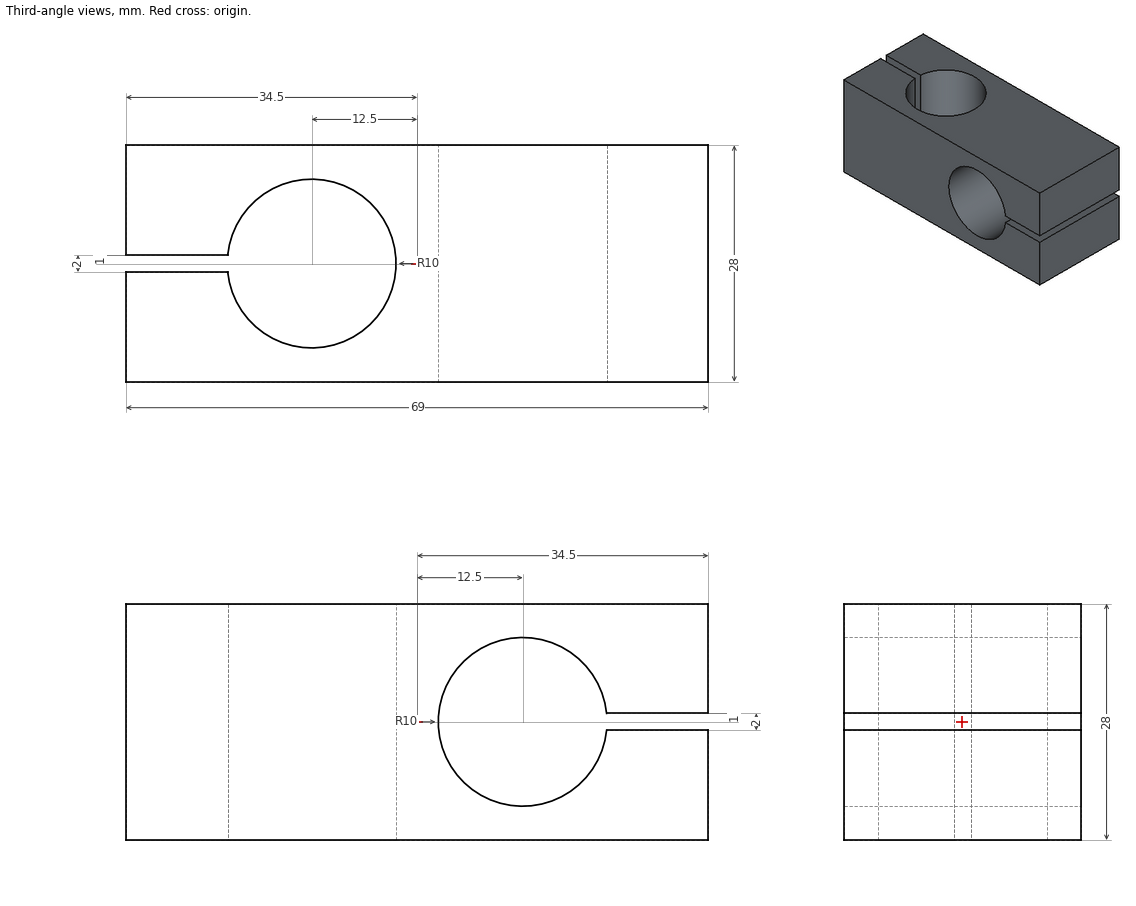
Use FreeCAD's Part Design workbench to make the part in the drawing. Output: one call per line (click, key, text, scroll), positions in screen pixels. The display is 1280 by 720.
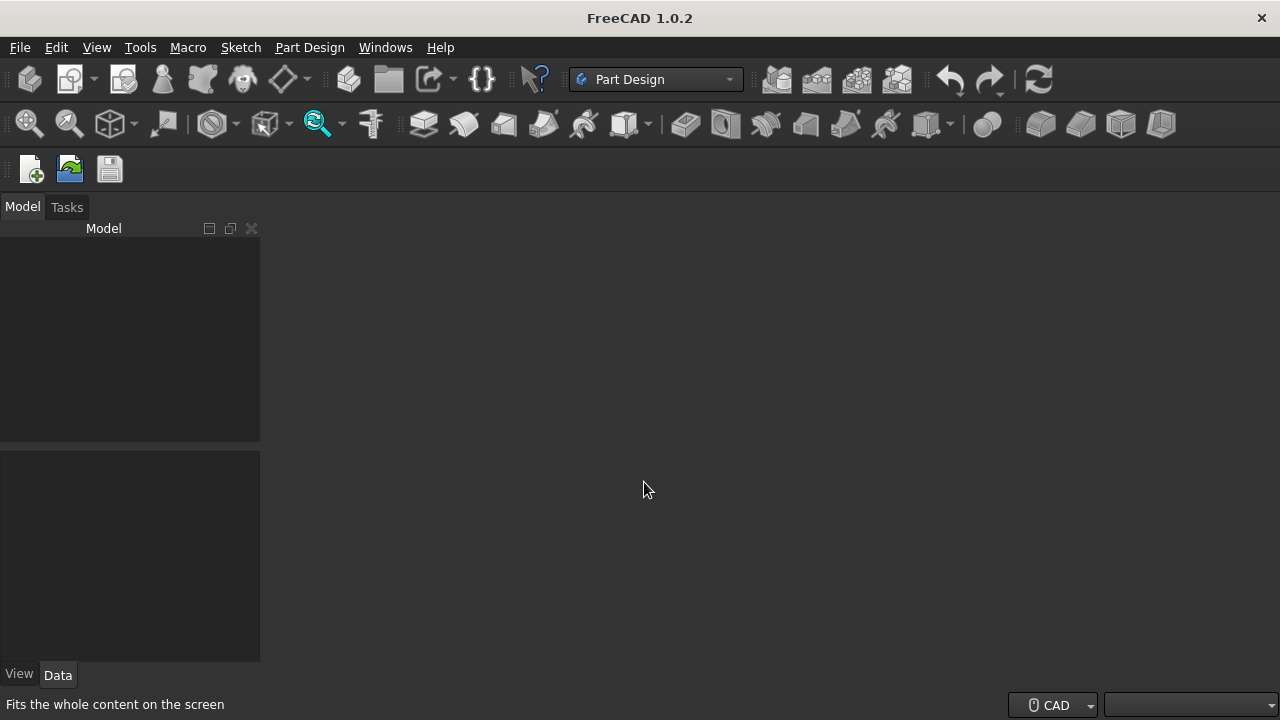
key(ctrl+n)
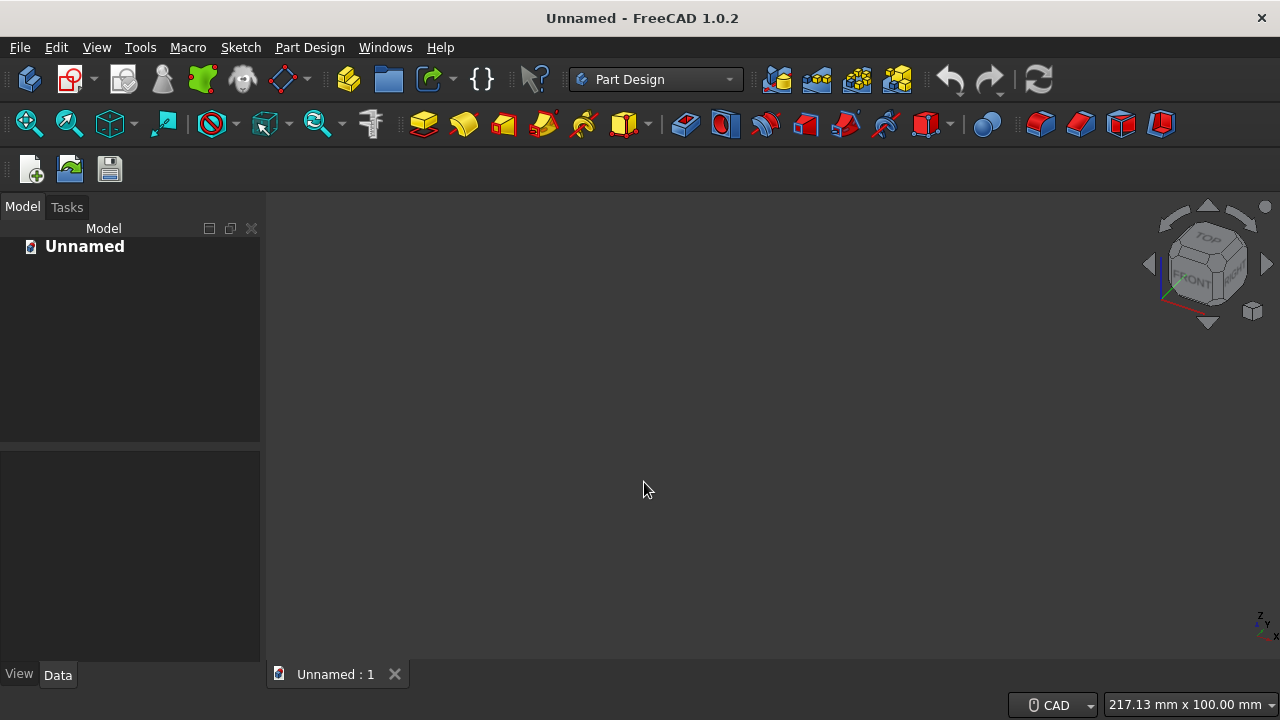
click(70, 80)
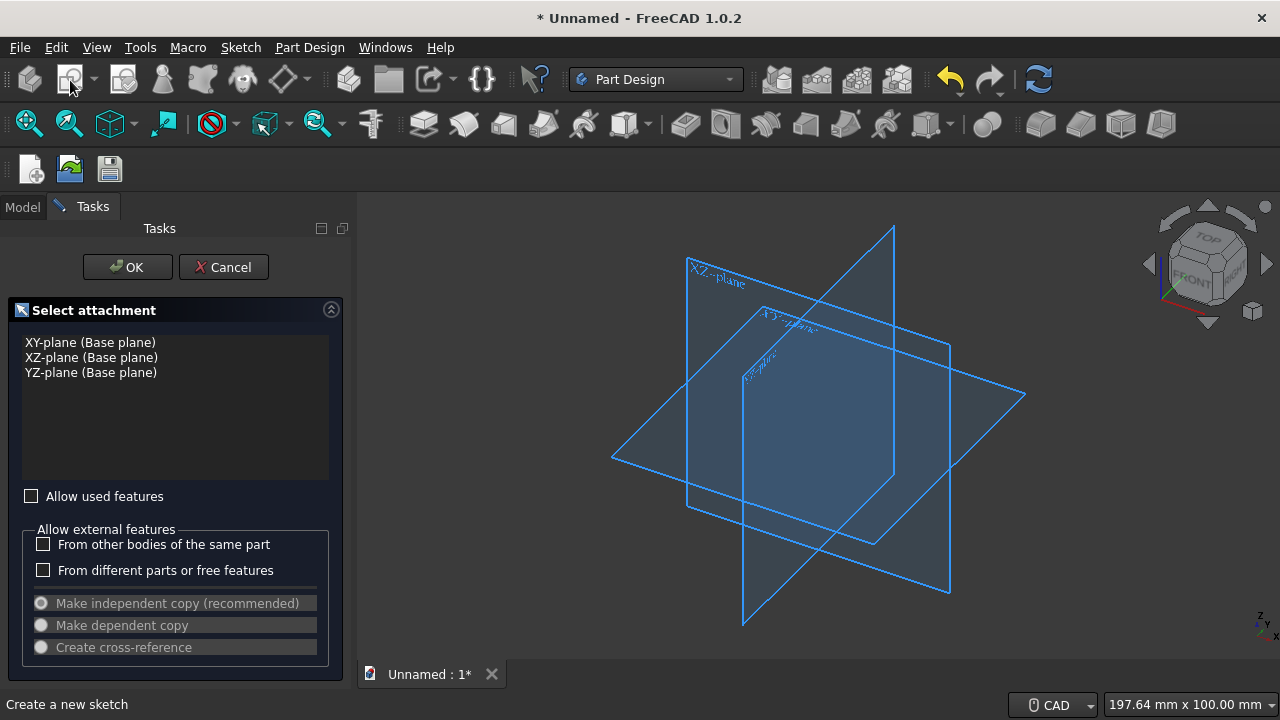
click(82, 342)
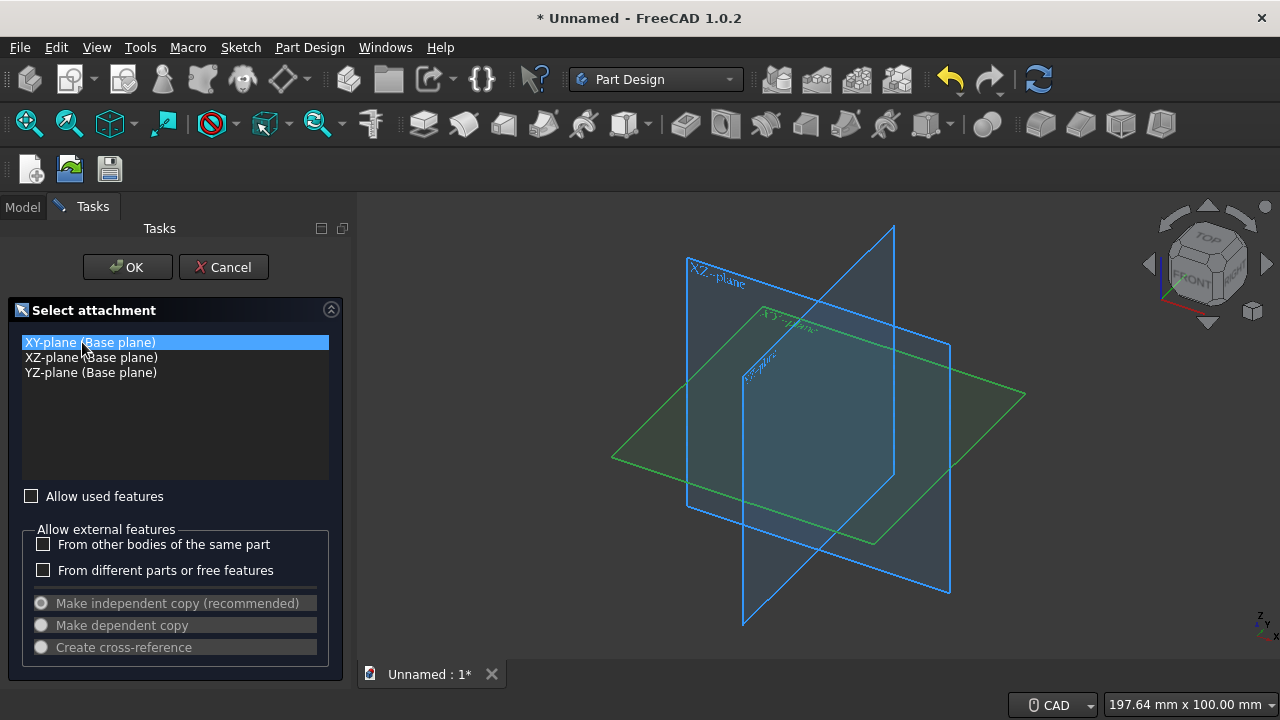
click(128, 267)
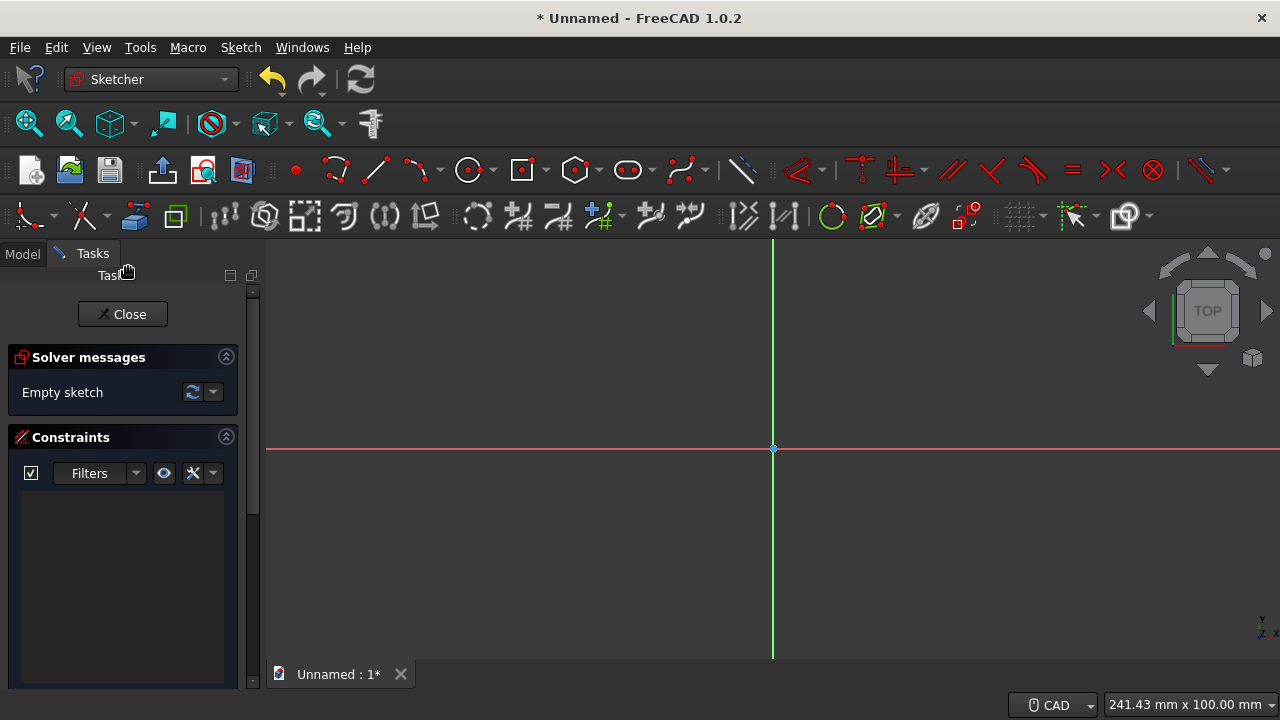
scroll(856, 449, up, 3)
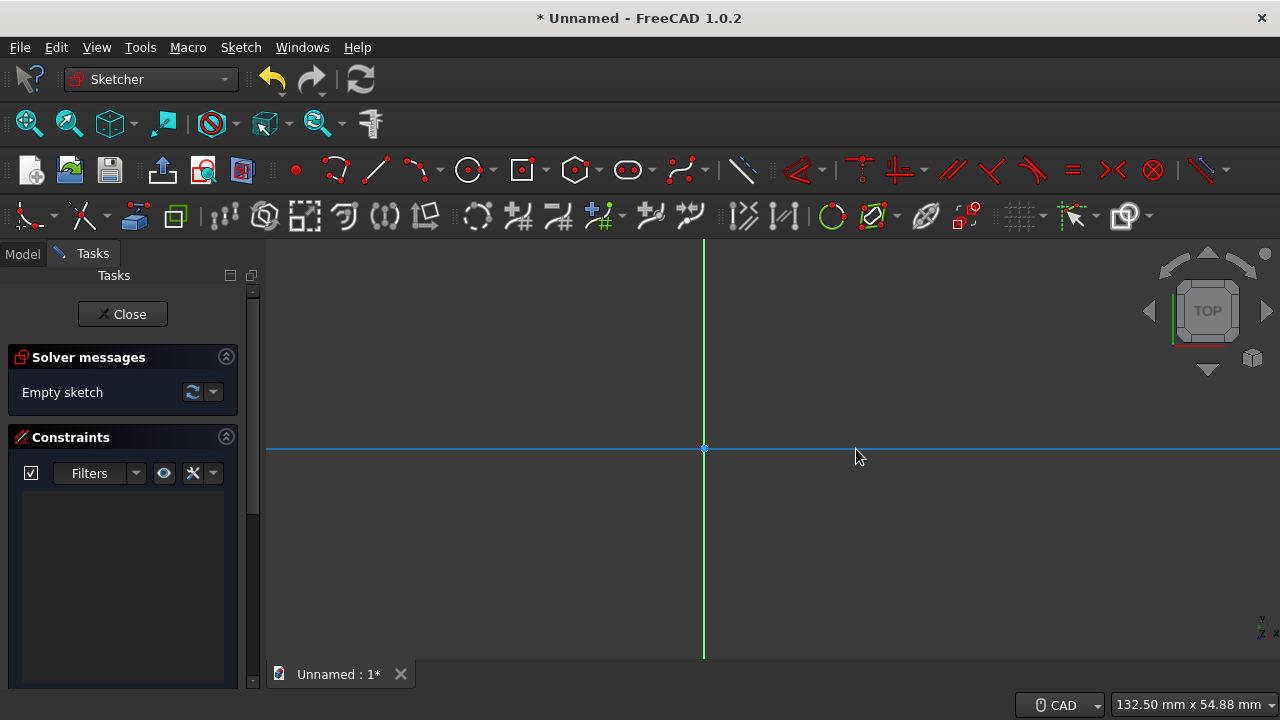
click(522, 170)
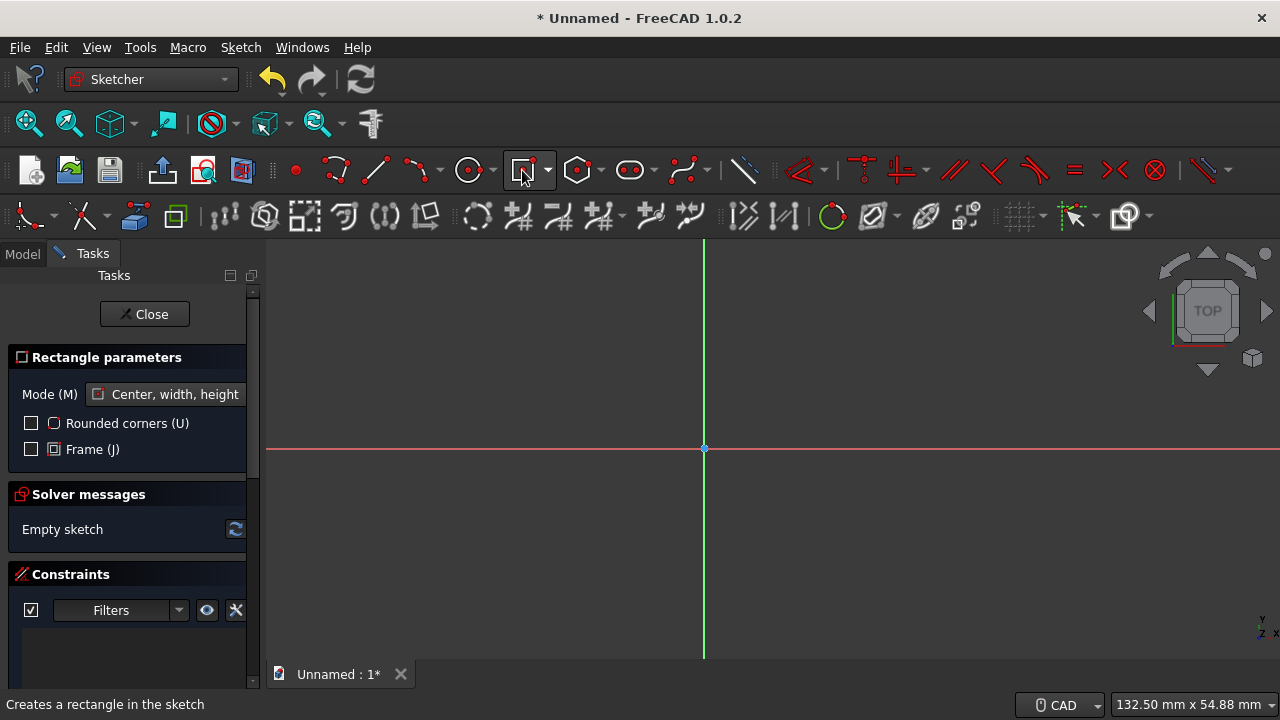
click(704, 449)
move(968, 341)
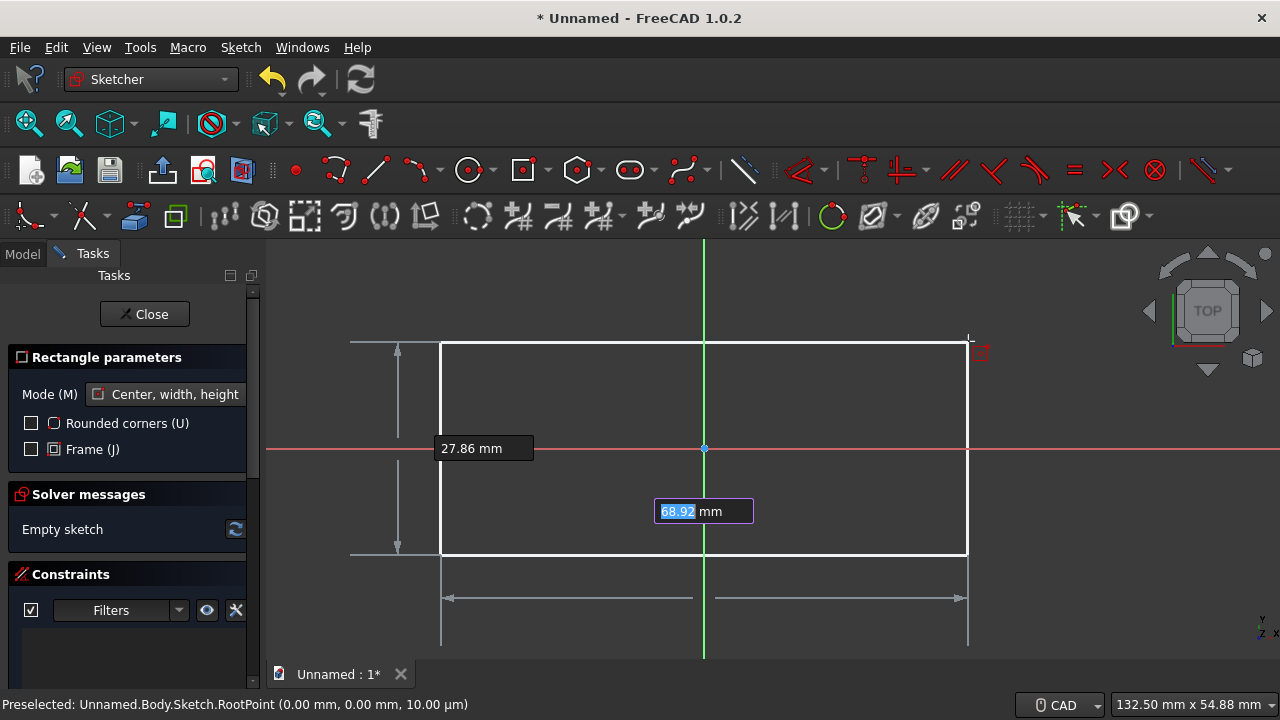
text(69)
key(Tab)
text(28)
key(Return)
key(Escape)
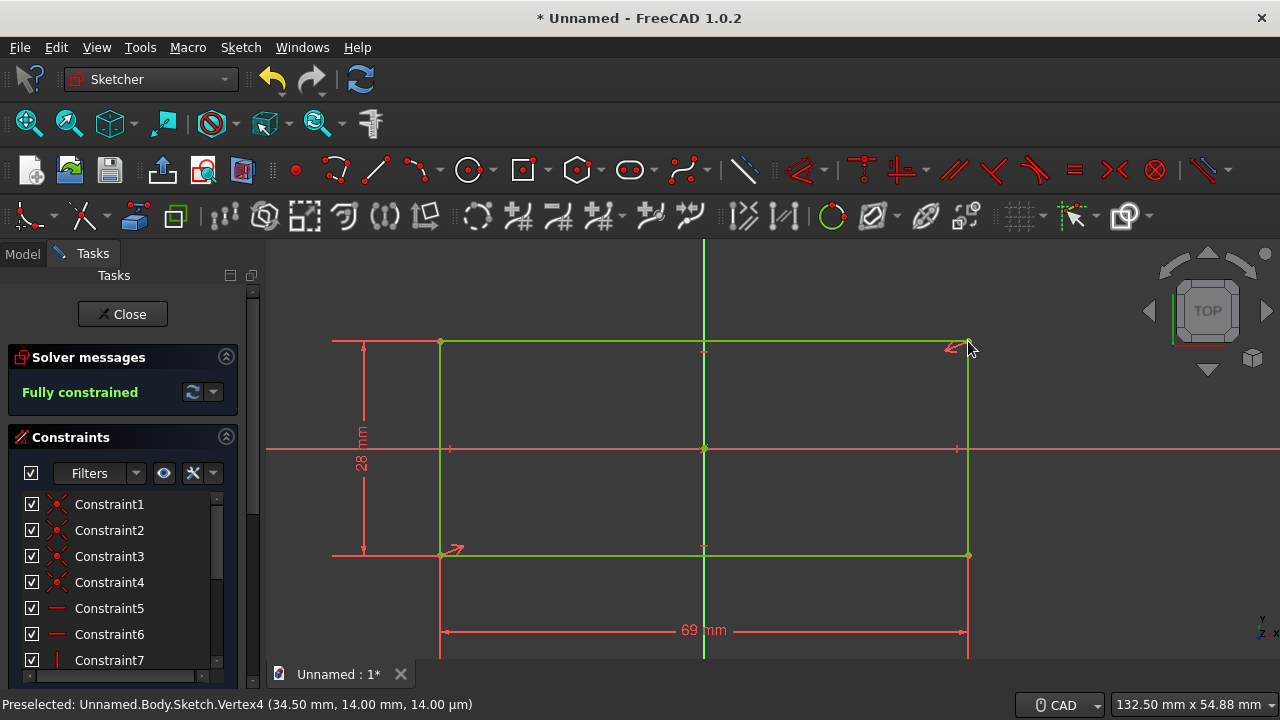
click(123, 314)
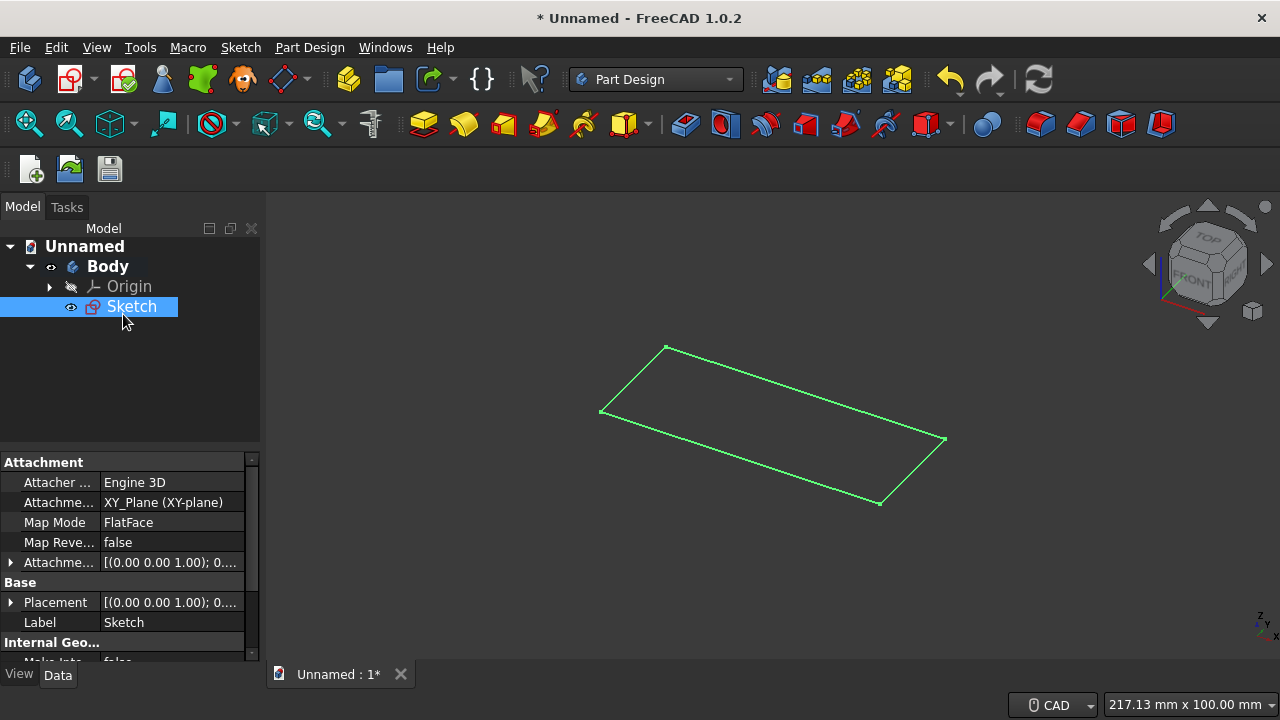
click(424, 124)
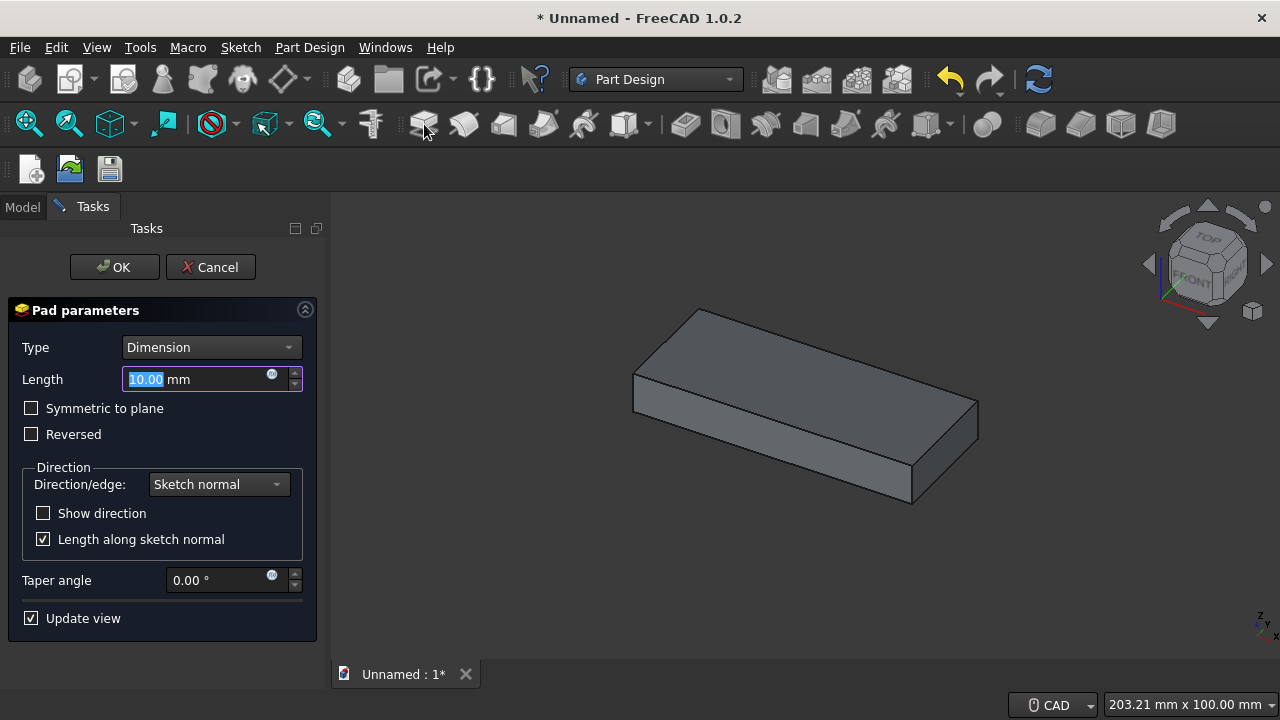
text(28)
key(Tab)